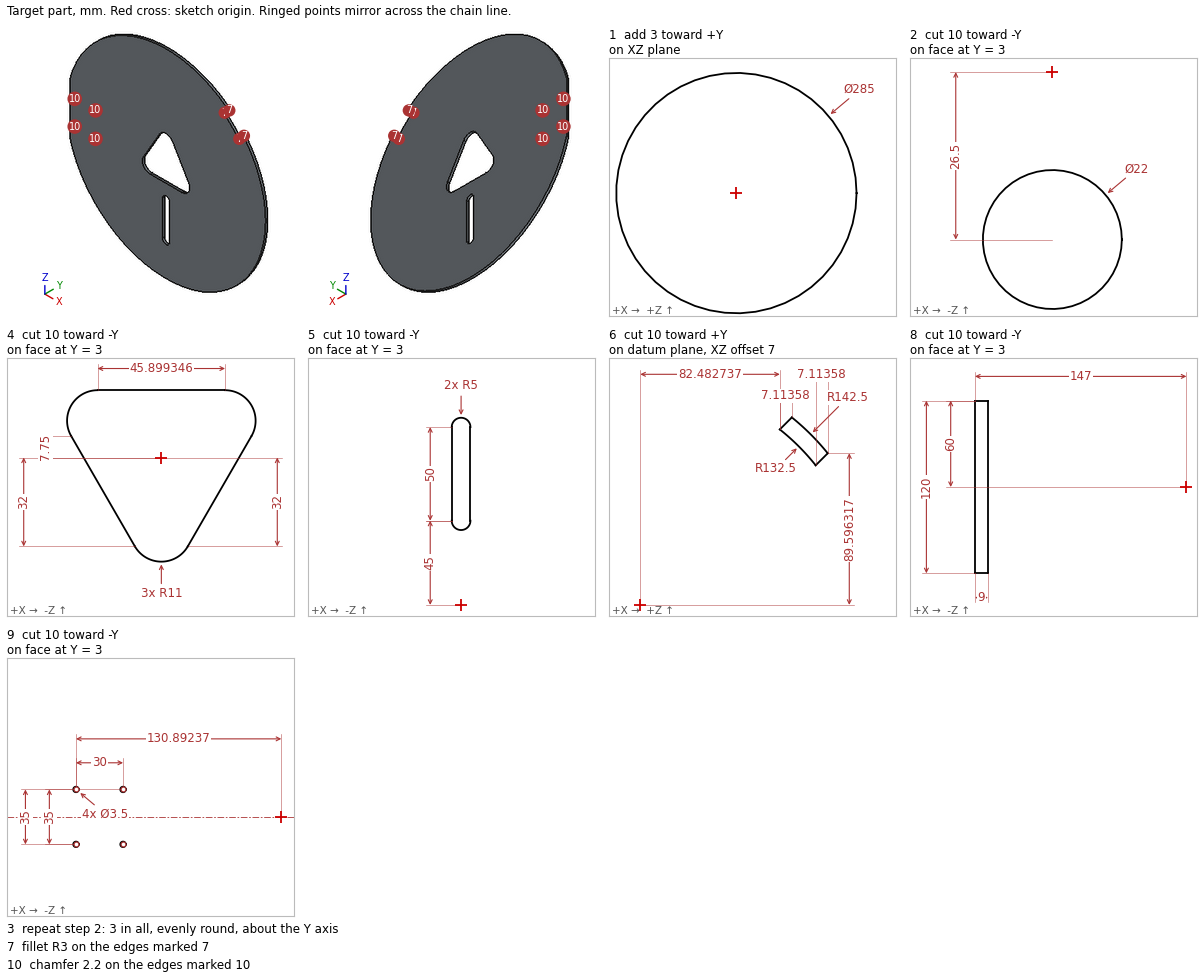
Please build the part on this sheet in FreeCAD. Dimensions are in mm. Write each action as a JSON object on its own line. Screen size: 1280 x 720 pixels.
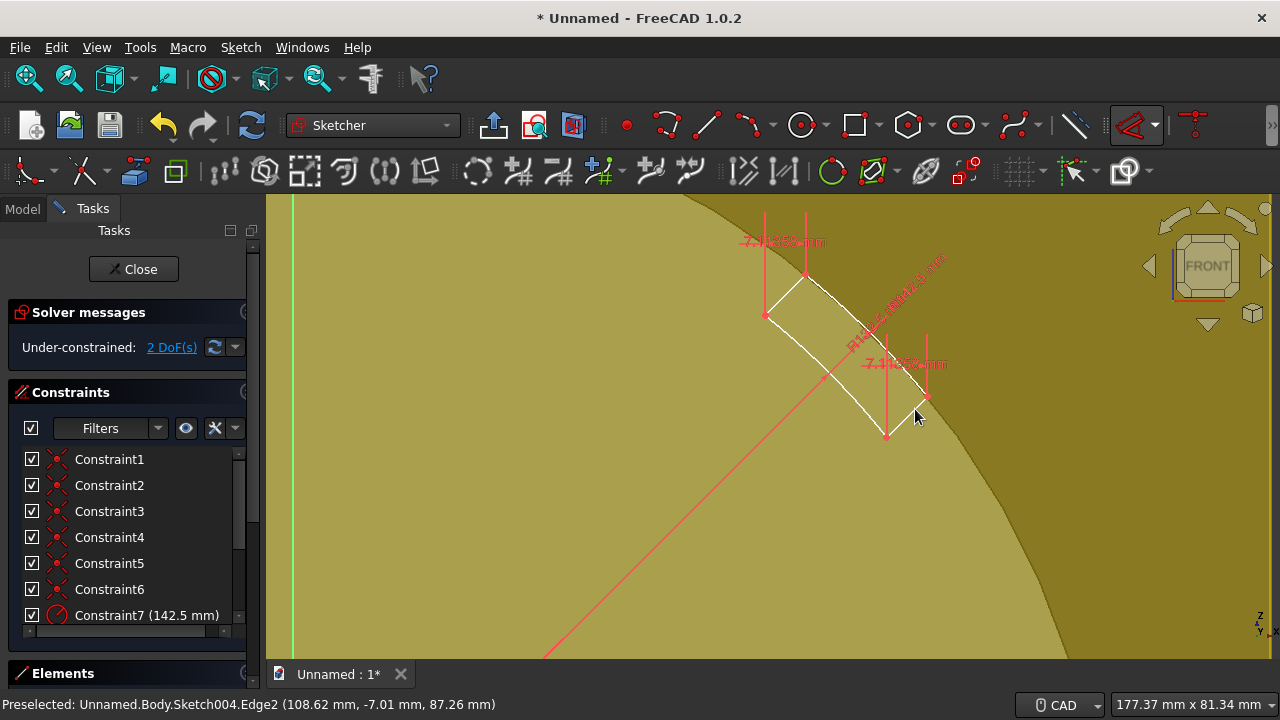
{"action": "left_click", "coordinate": [765, 316]}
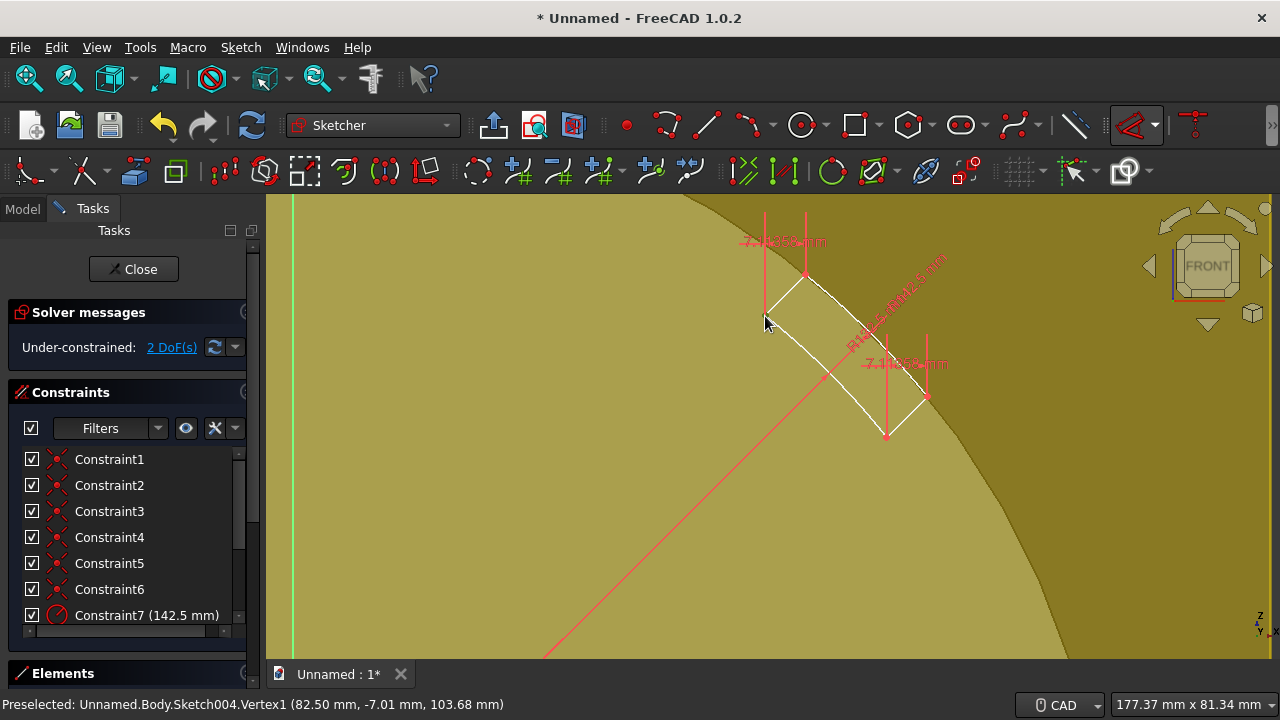
{"action": "left_click", "coordinate": [1158, 126]}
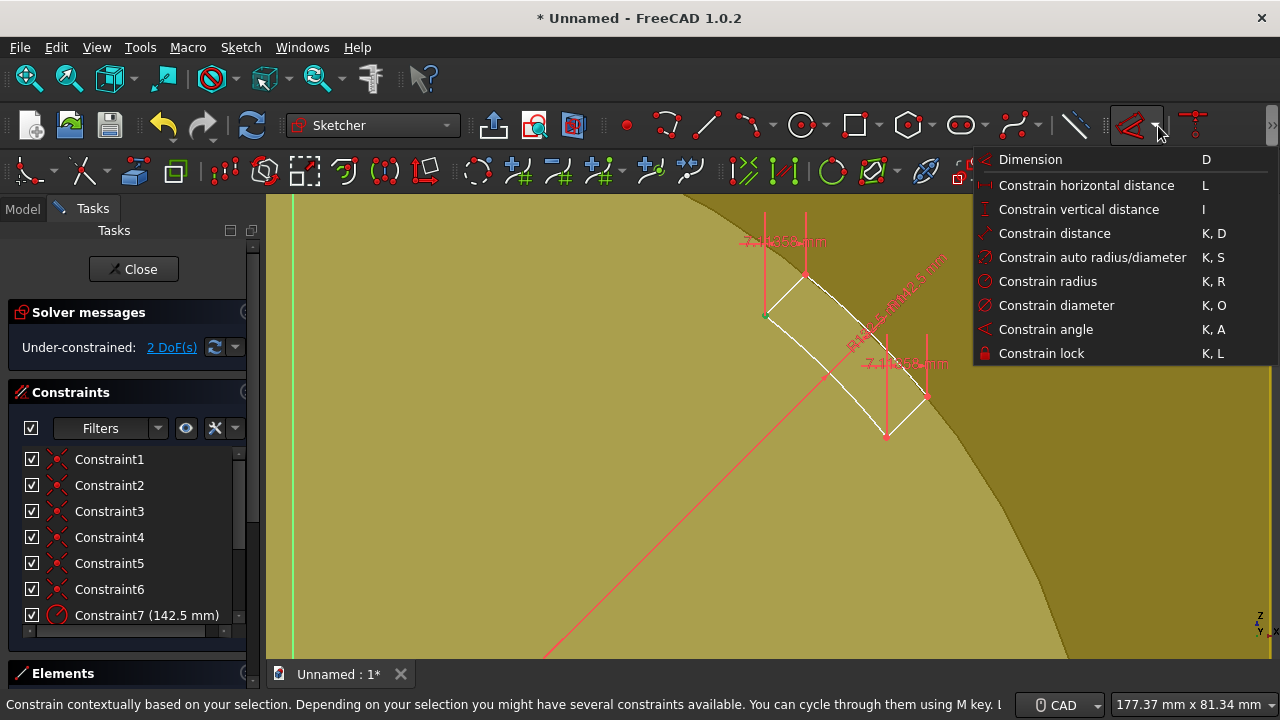
{"action": "left_click", "coordinate": [1126, 185]}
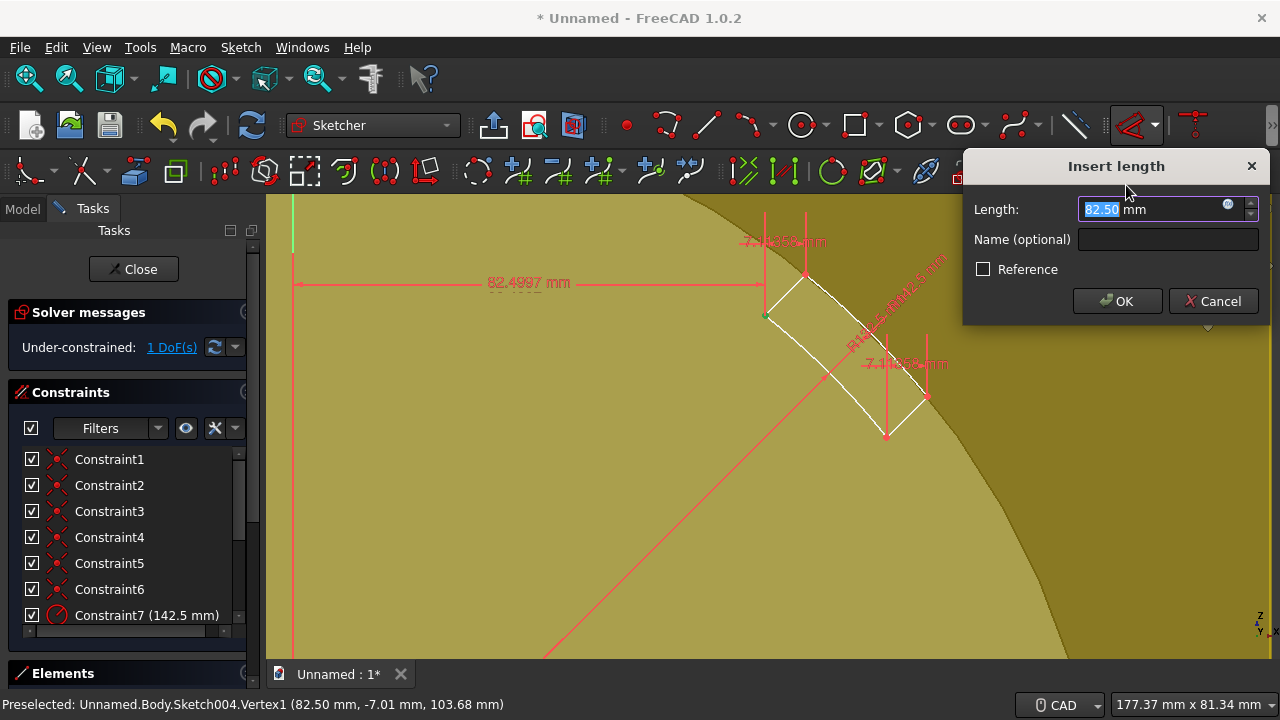
{"action": "type", "text": "82.482737"}
{"action": "key", "text": "Return"}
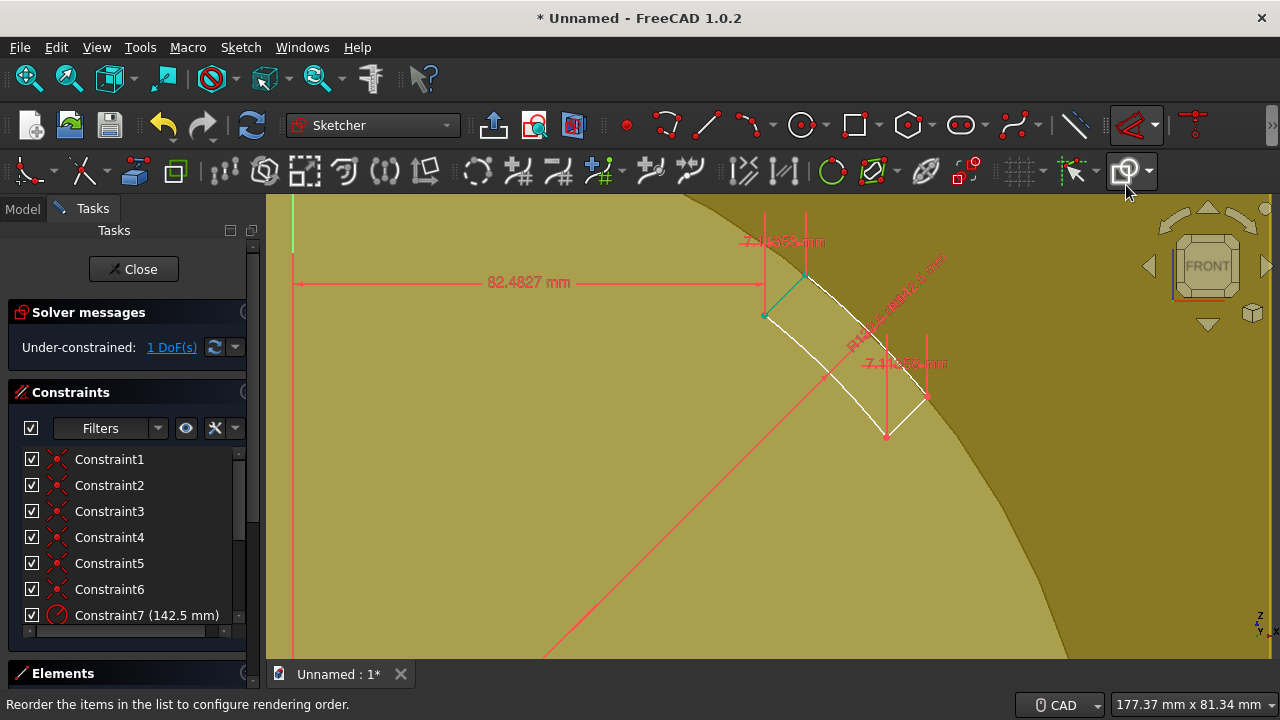
{"action": "left_click", "coordinate": [927, 397]}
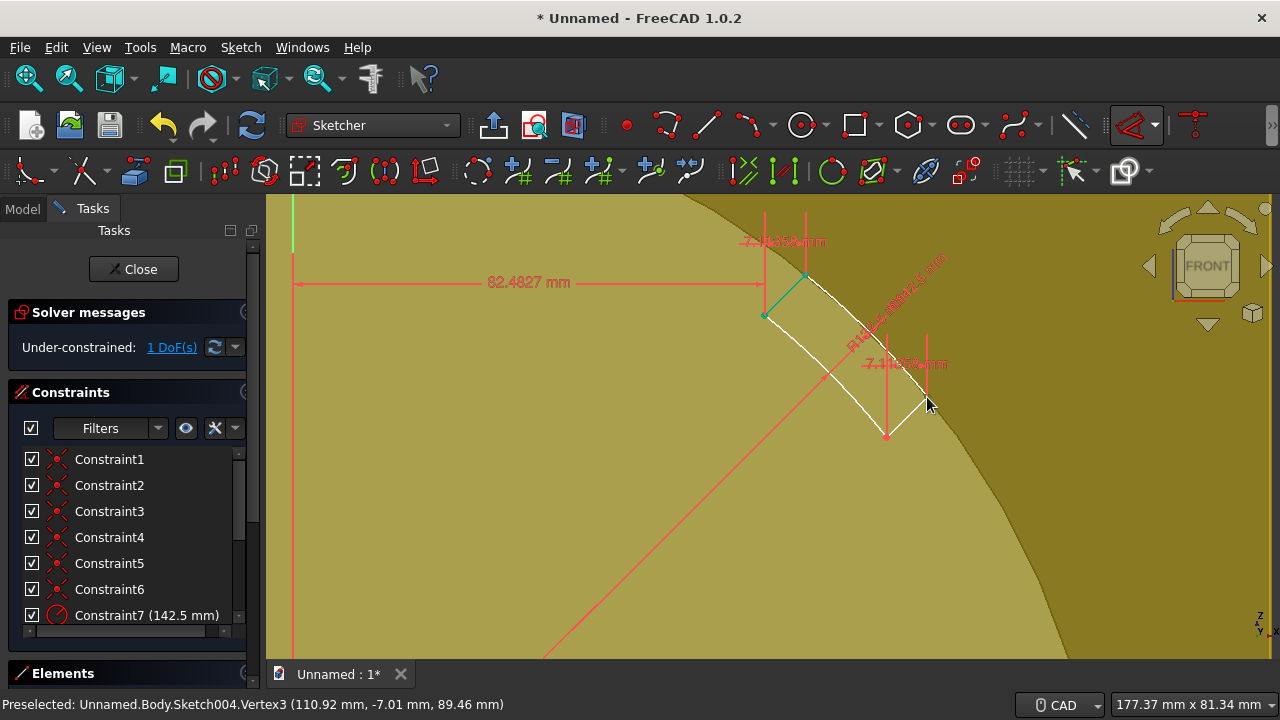
{"action": "key", "text": "i"}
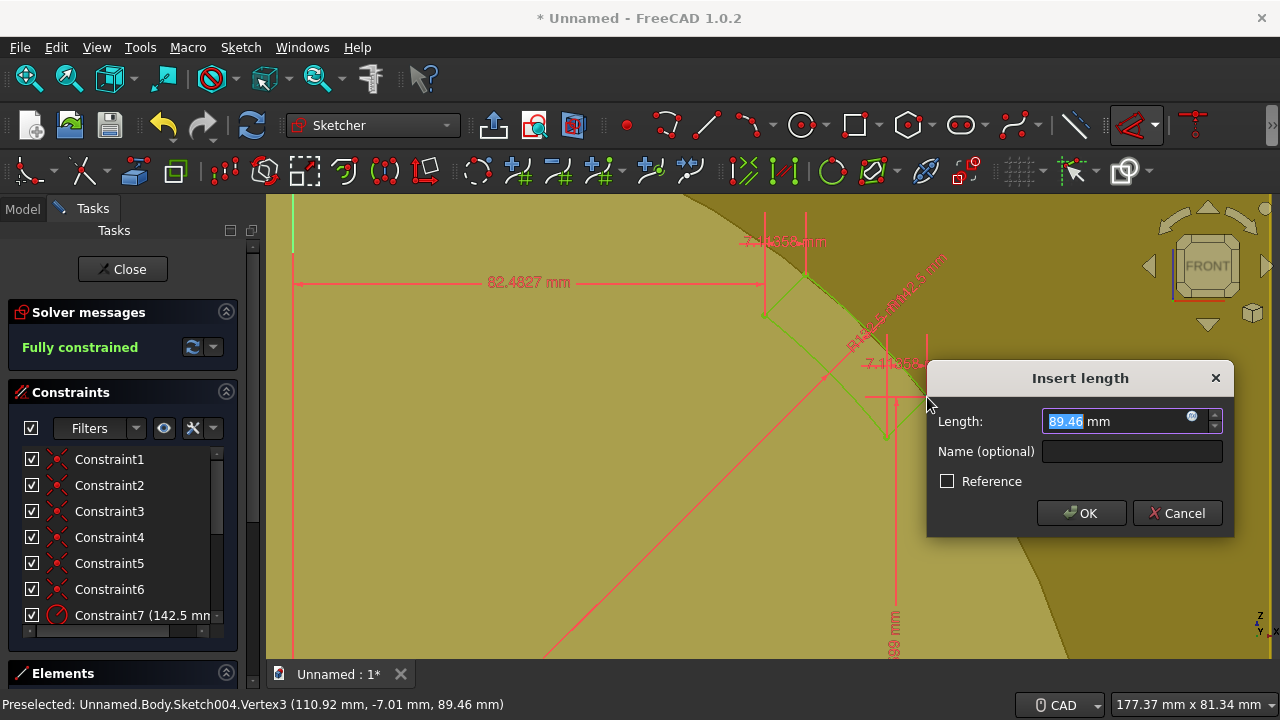
{"action": "type", "text": "89.596317"}
{"action": "key", "text": "Return"}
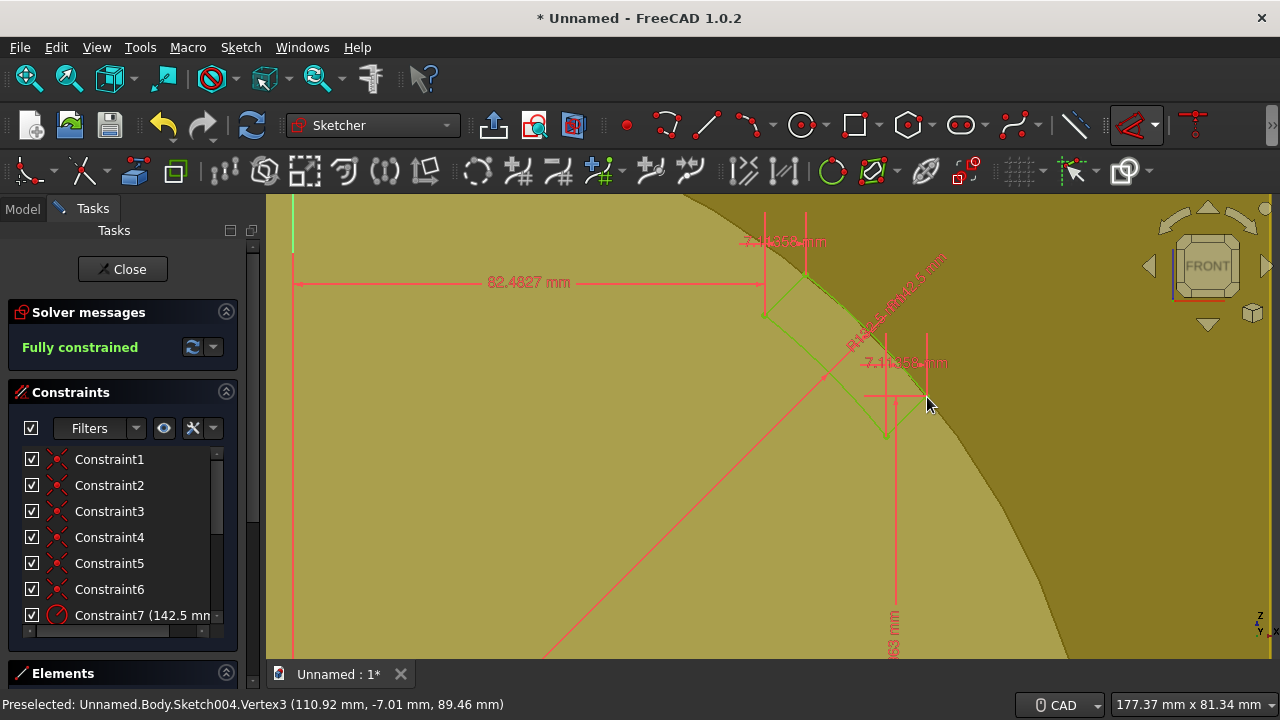
{"action": "left_click", "coordinate": [123, 269]}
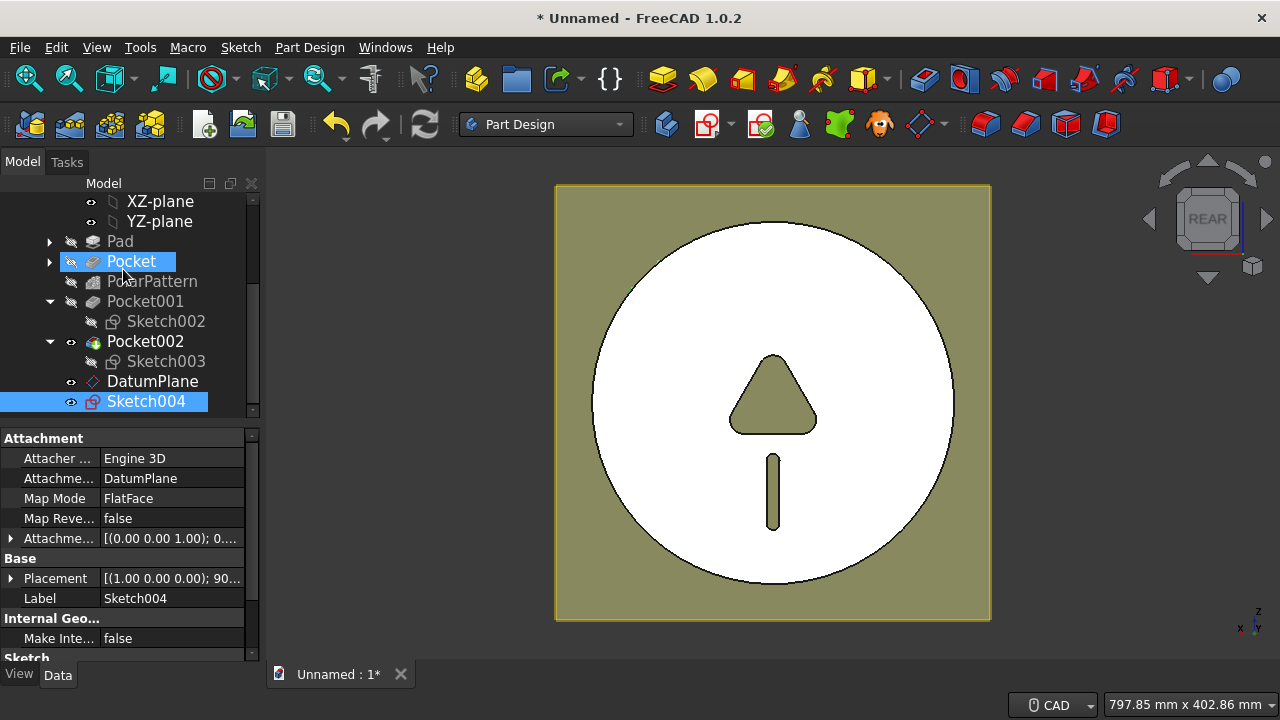
{"action": "left_click", "coordinate": [926, 80]}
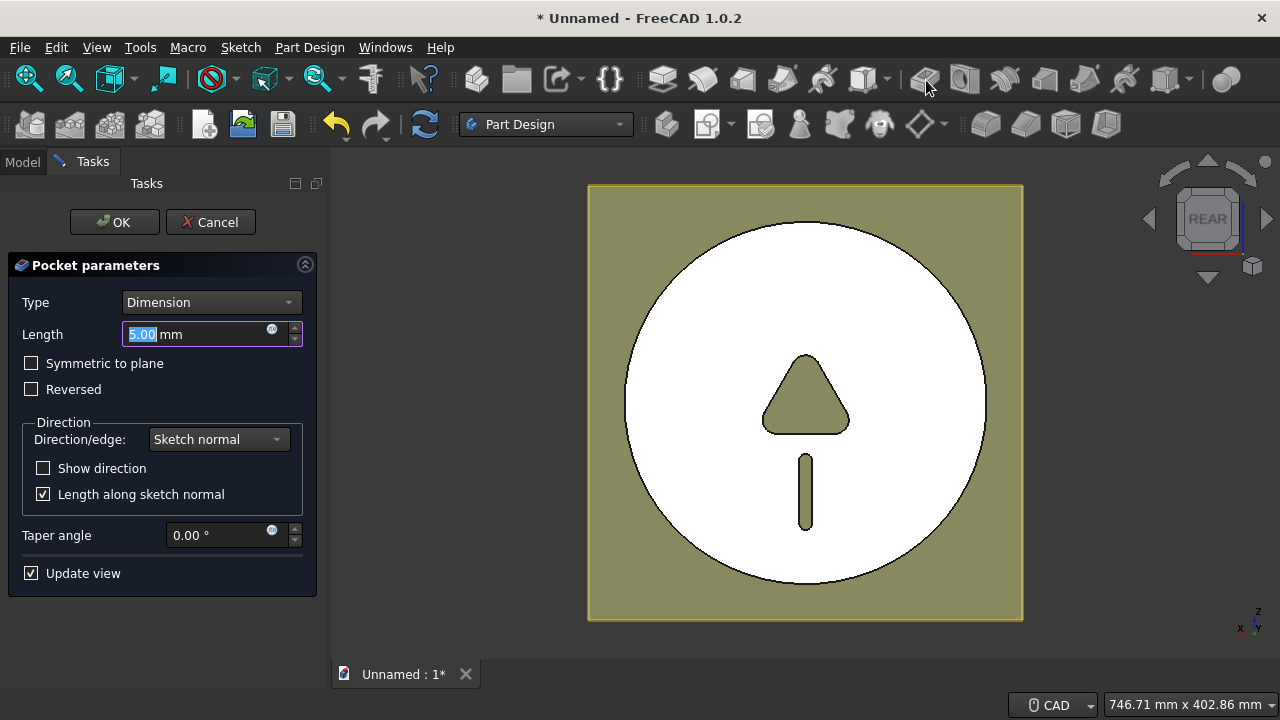
{"action": "type", "text": "10"}
{"action": "key", "text": "Tab"}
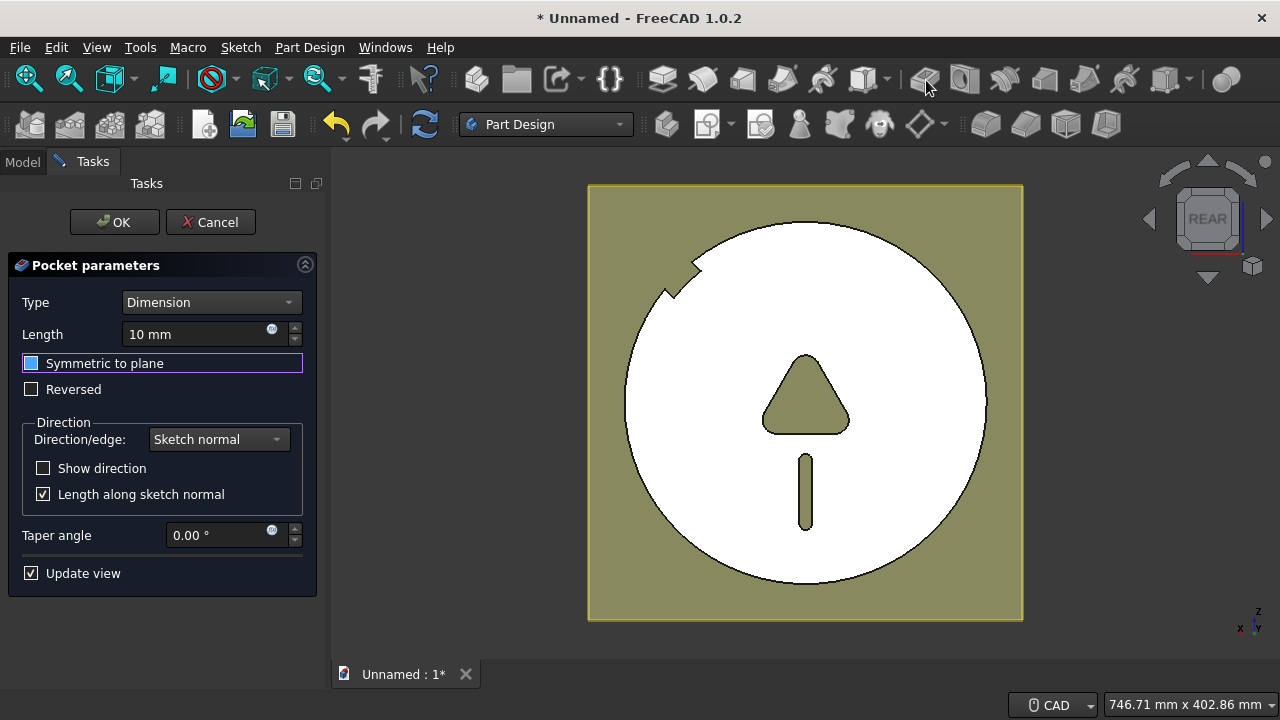
{"action": "left_click", "coordinate": [115, 222]}